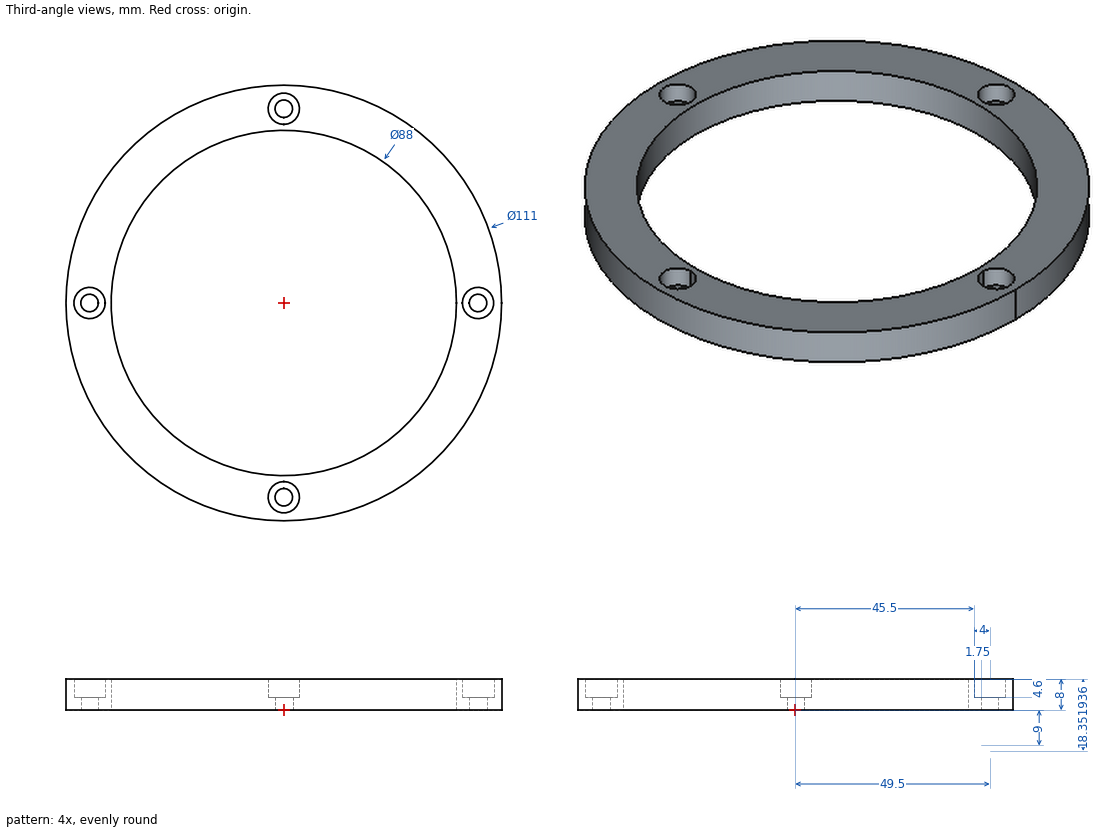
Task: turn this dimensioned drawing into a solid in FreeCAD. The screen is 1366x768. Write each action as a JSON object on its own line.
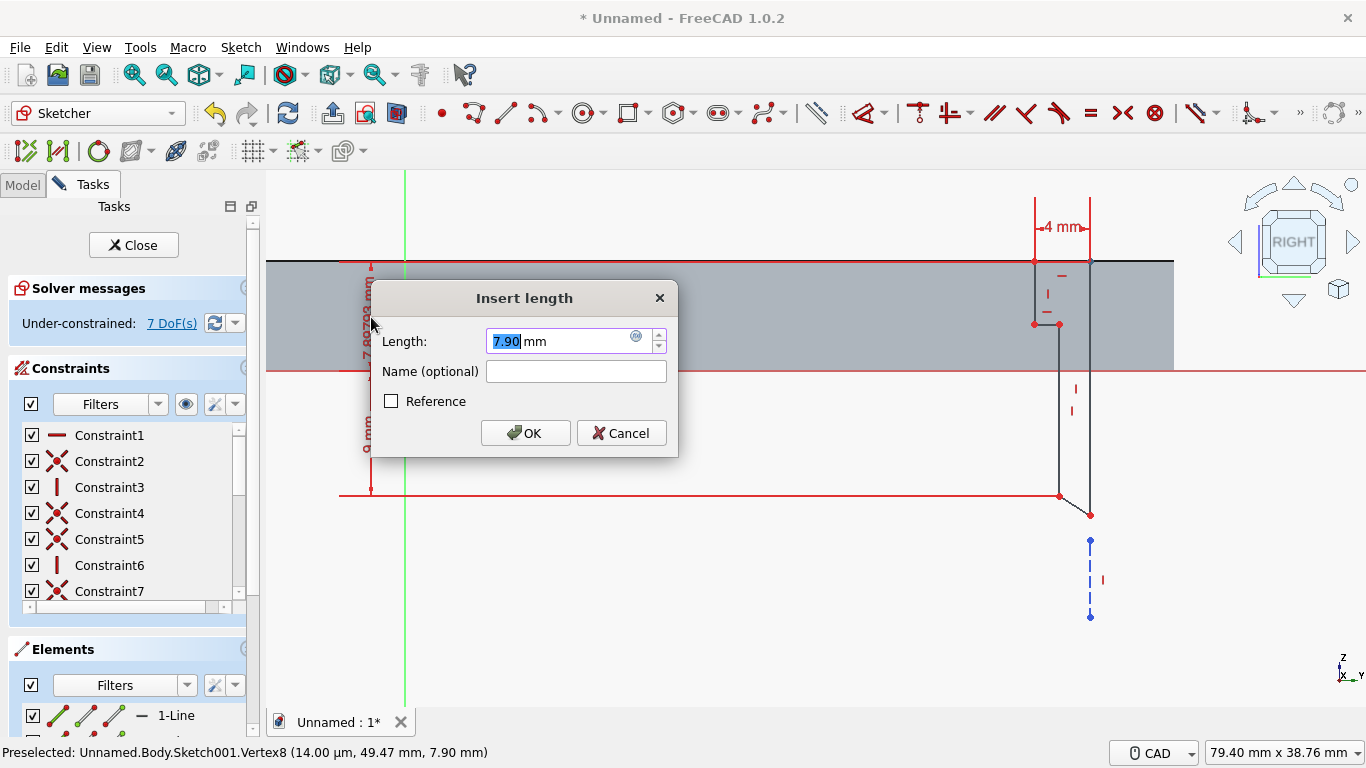
{"action": "type", "text": "8"}
{"action": "key", "text": "Return"}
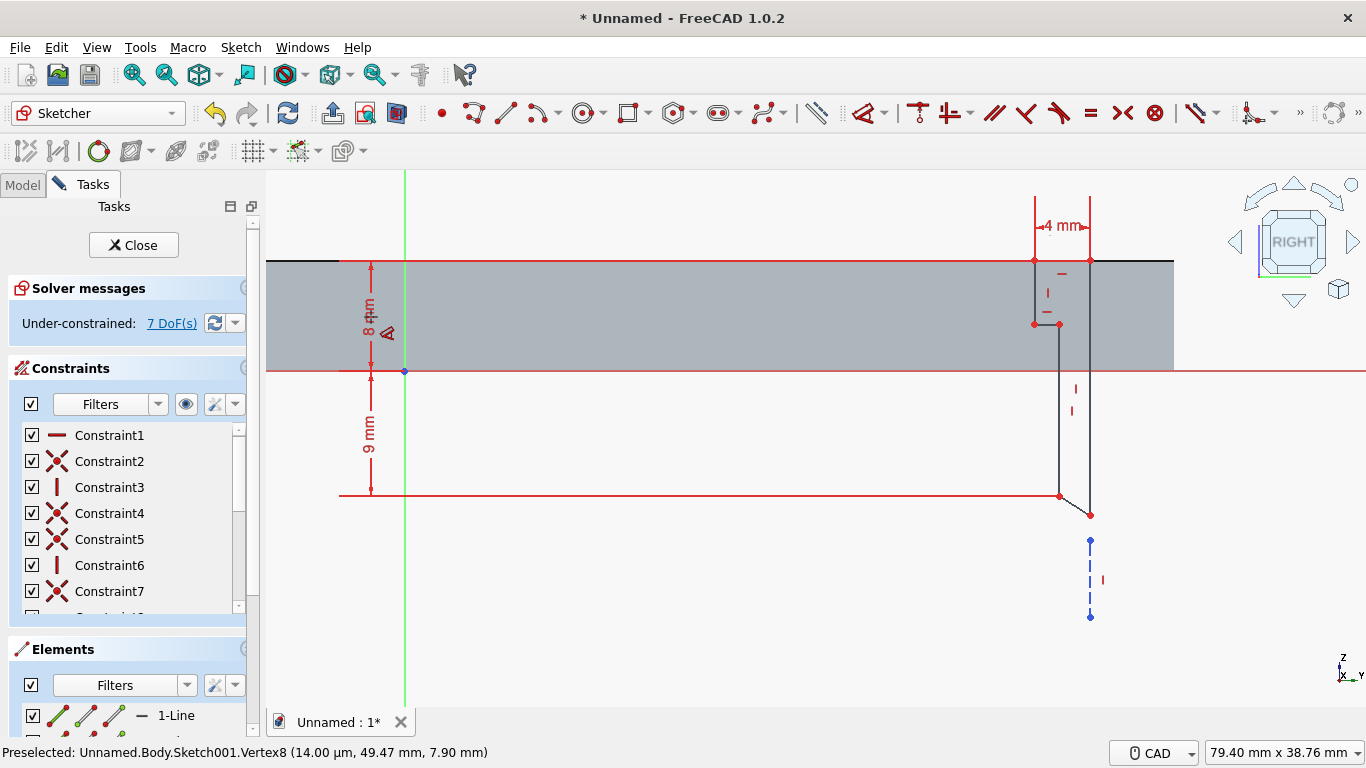
{"action": "left_click", "coordinate": [1035, 280]}
{"action": "left_click", "coordinate": [1069, 293]}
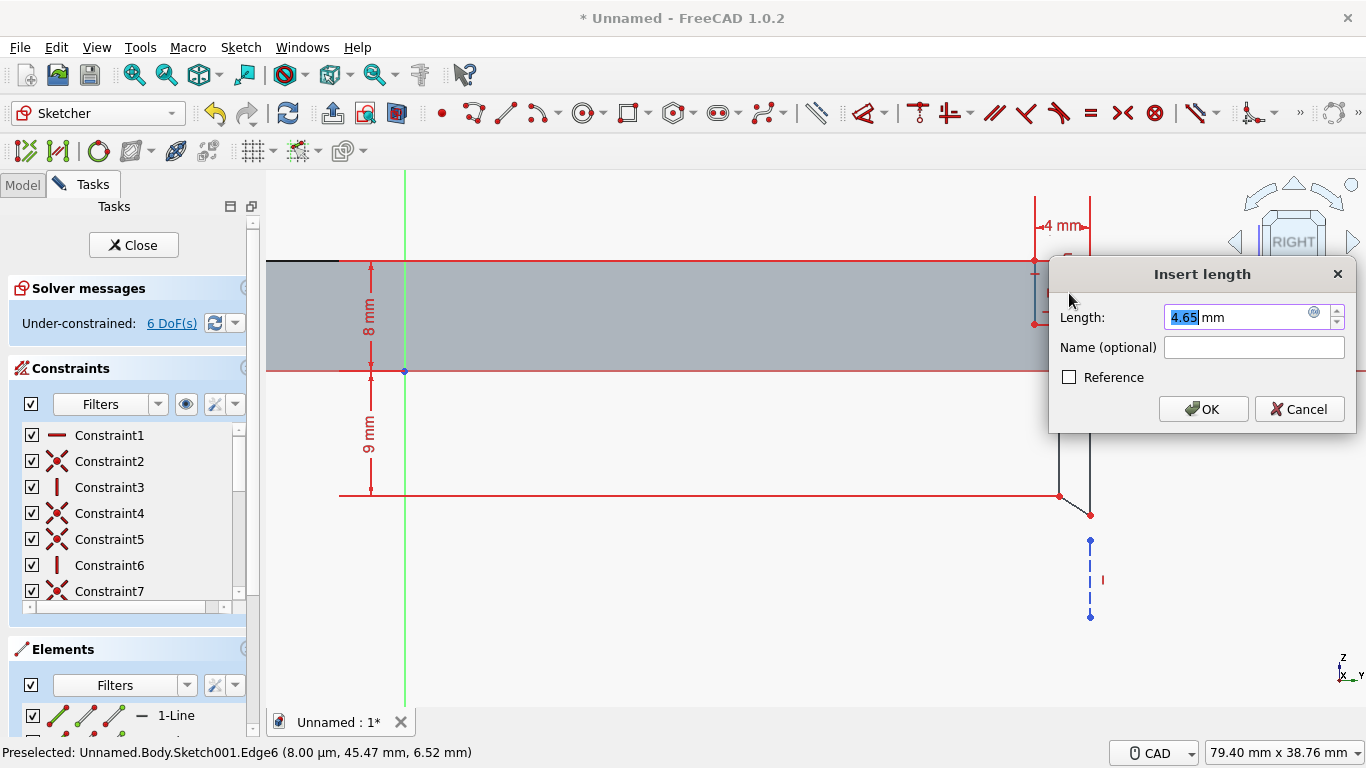
{"action": "type", "text": "4.6"}
{"action": "key", "text": "Return"}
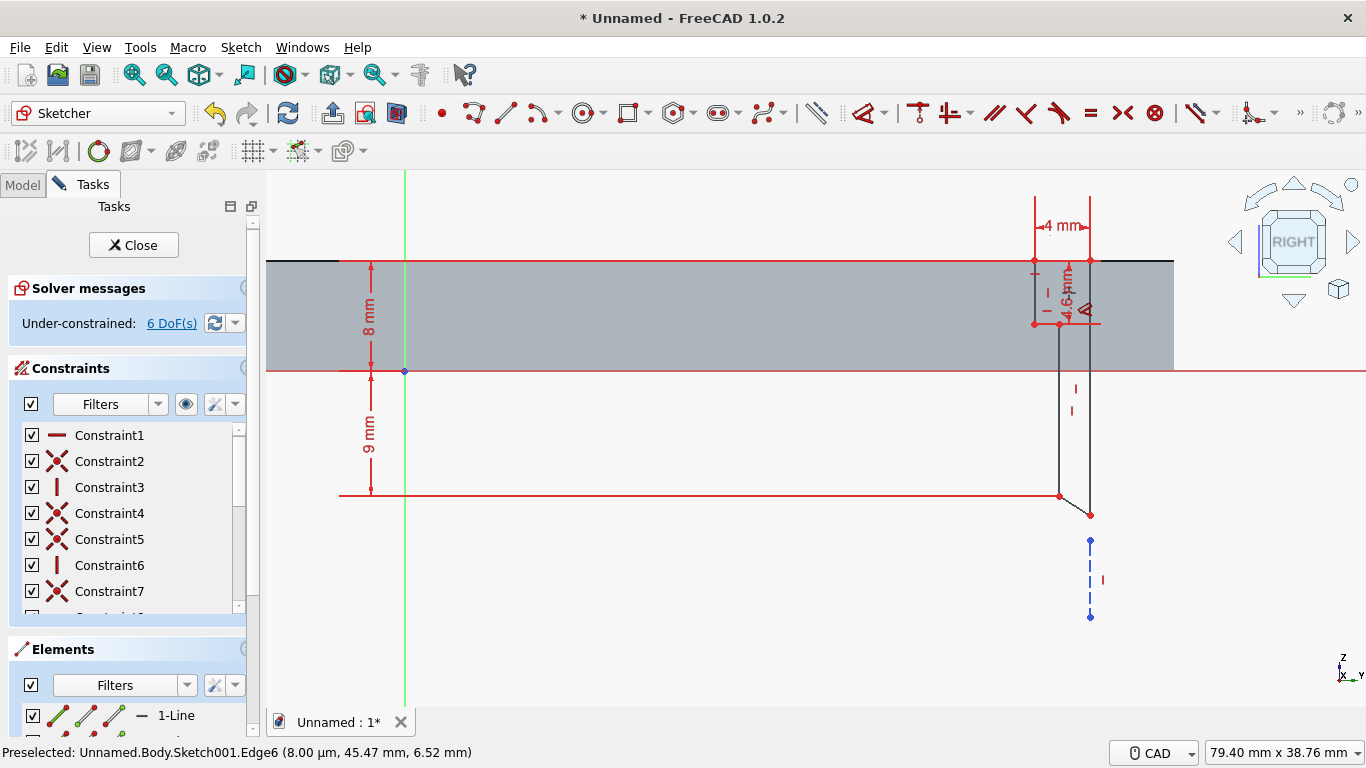
{"action": "scroll", "coordinate": [1045, 324], "scroll_direction": "up", "scroll_amount": 3}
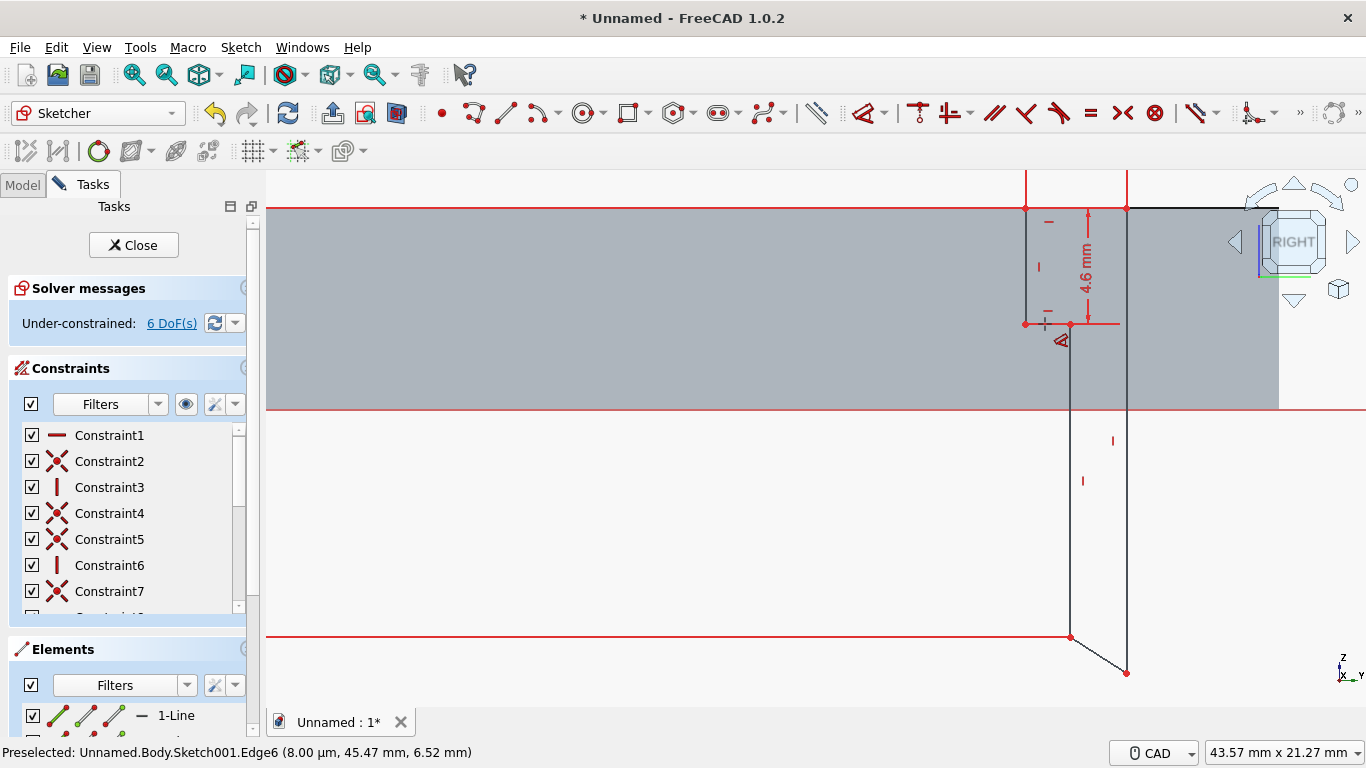
{"action": "left_click", "coordinate": [1044, 324]}
{"action": "left_click", "coordinate": [1048, 290]}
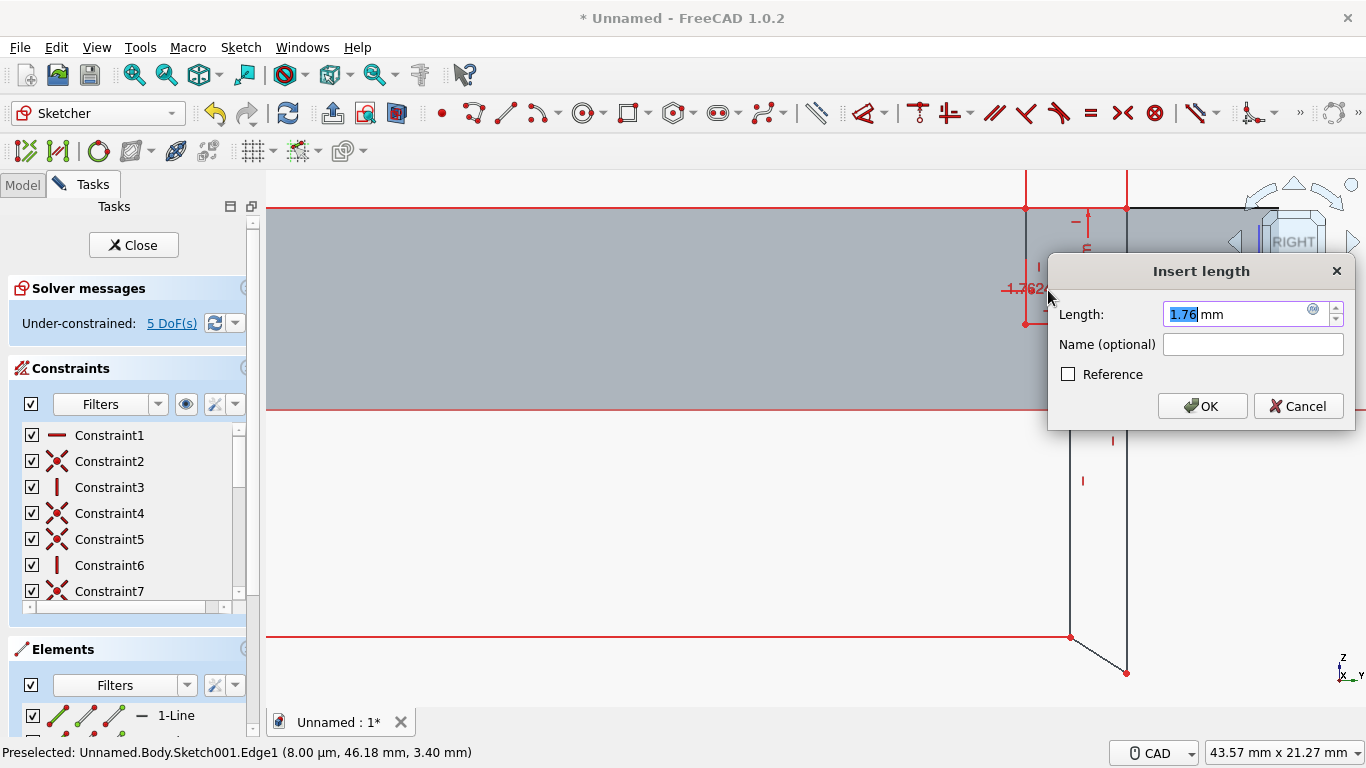
{"action": "type", "text": "1.75"}
{"action": "key", "text": "Return"}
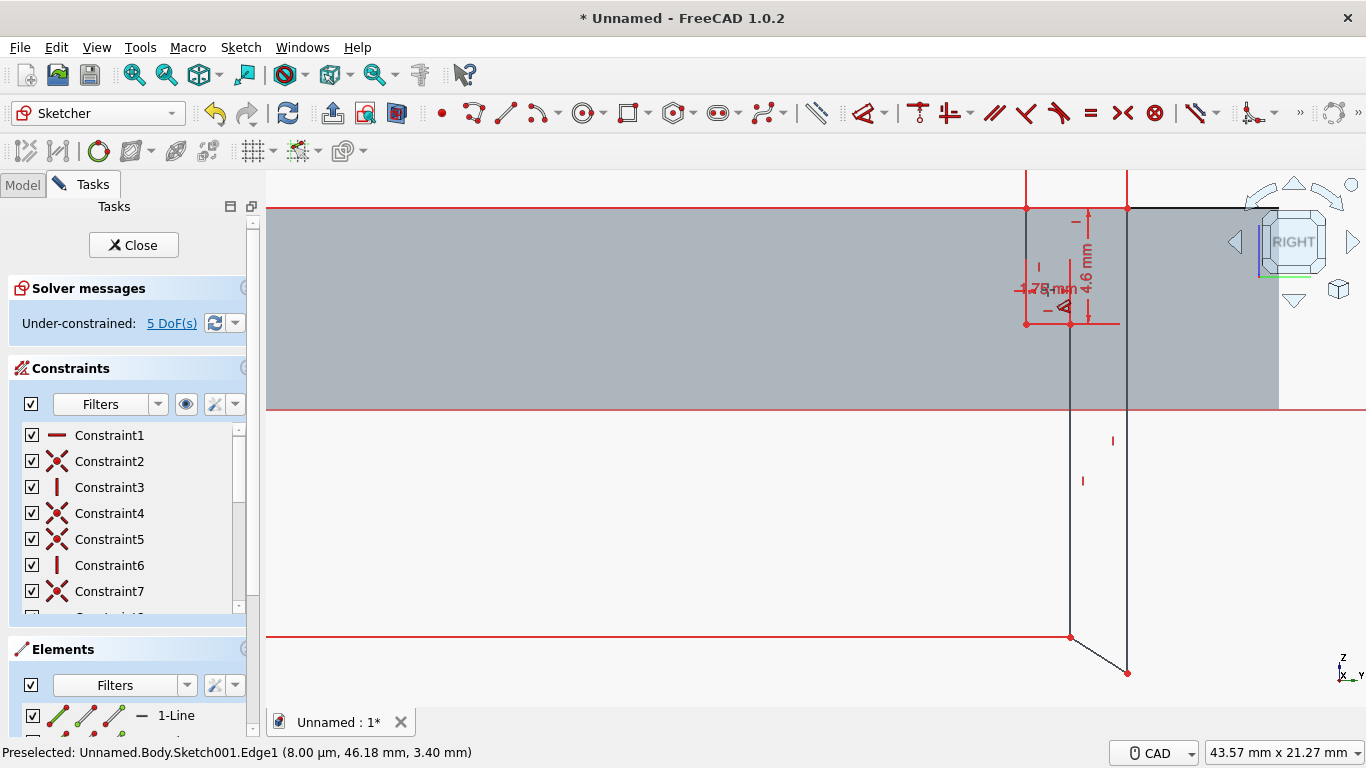
{"action": "left_click", "coordinate": [1026, 324]}
{"action": "left_click", "coordinate": [660, 290]}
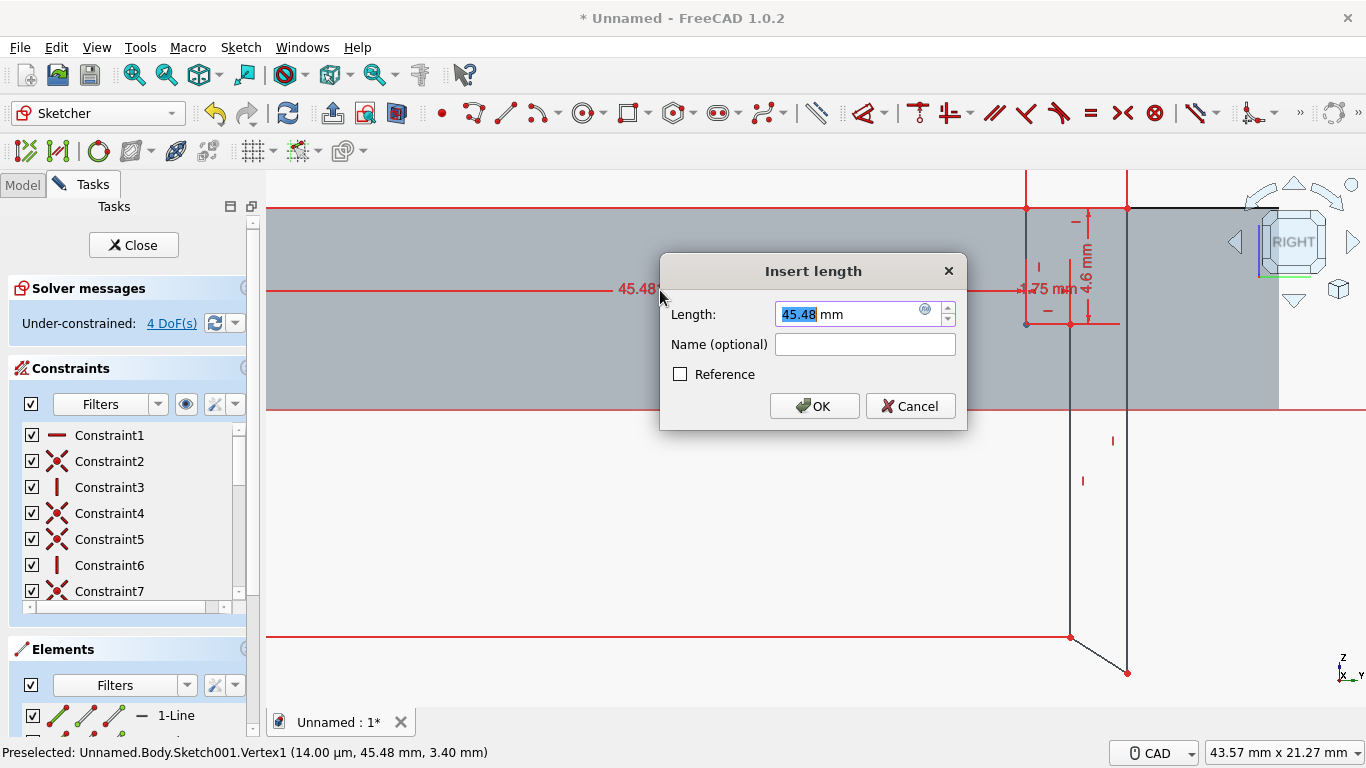
{"action": "type", "text": "45.5"}
{"action": "key", "text": "Return"}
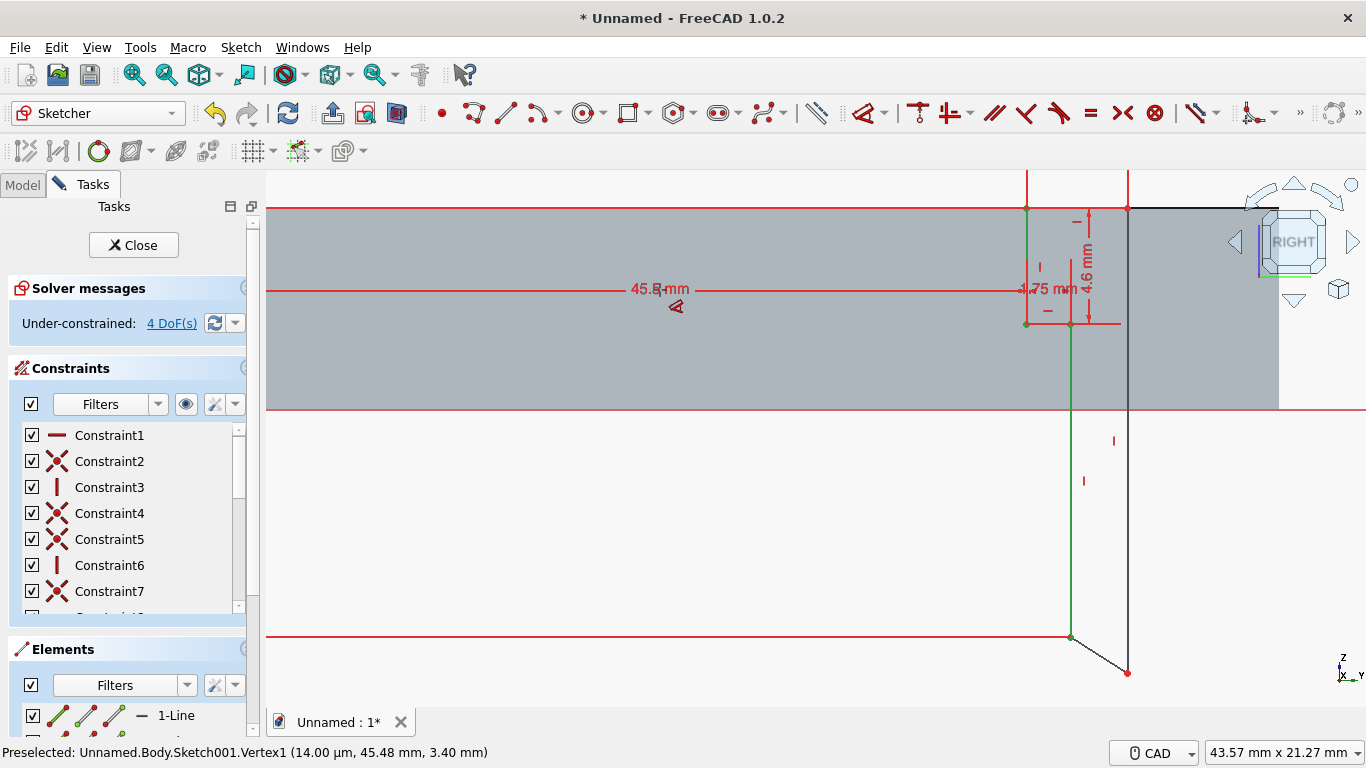
{"action": "scroll", "coordinate": [1045, 324], "scroll_direction": "down", "scroll_amount": 3}